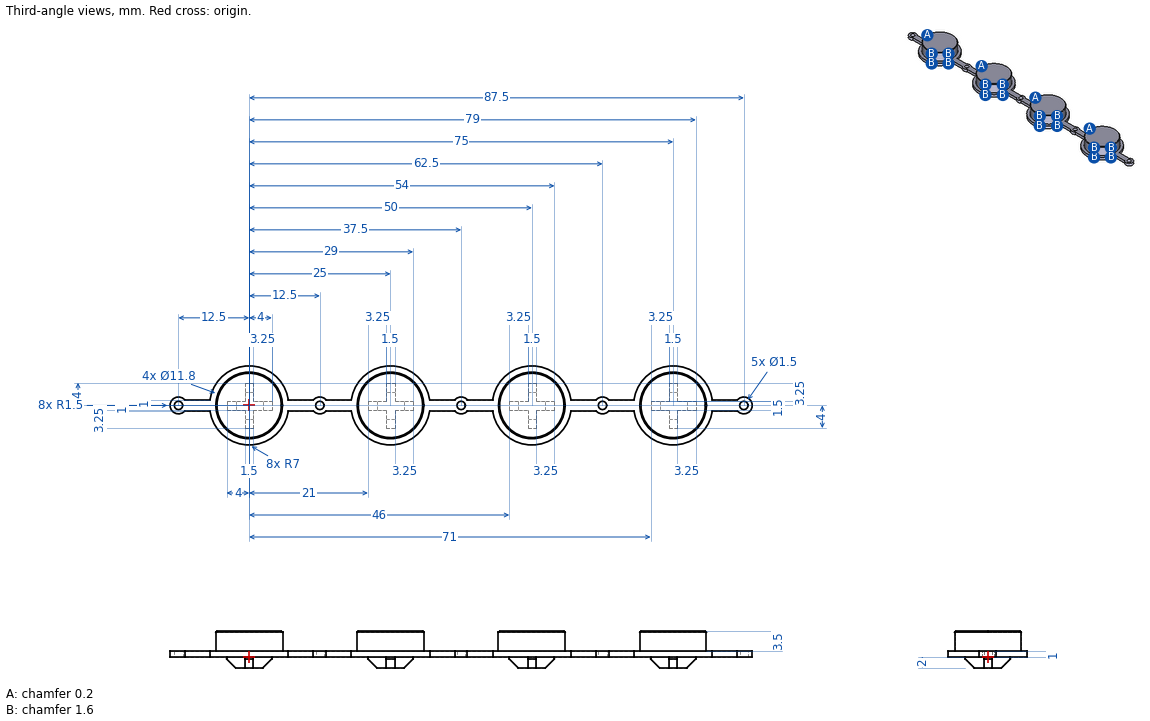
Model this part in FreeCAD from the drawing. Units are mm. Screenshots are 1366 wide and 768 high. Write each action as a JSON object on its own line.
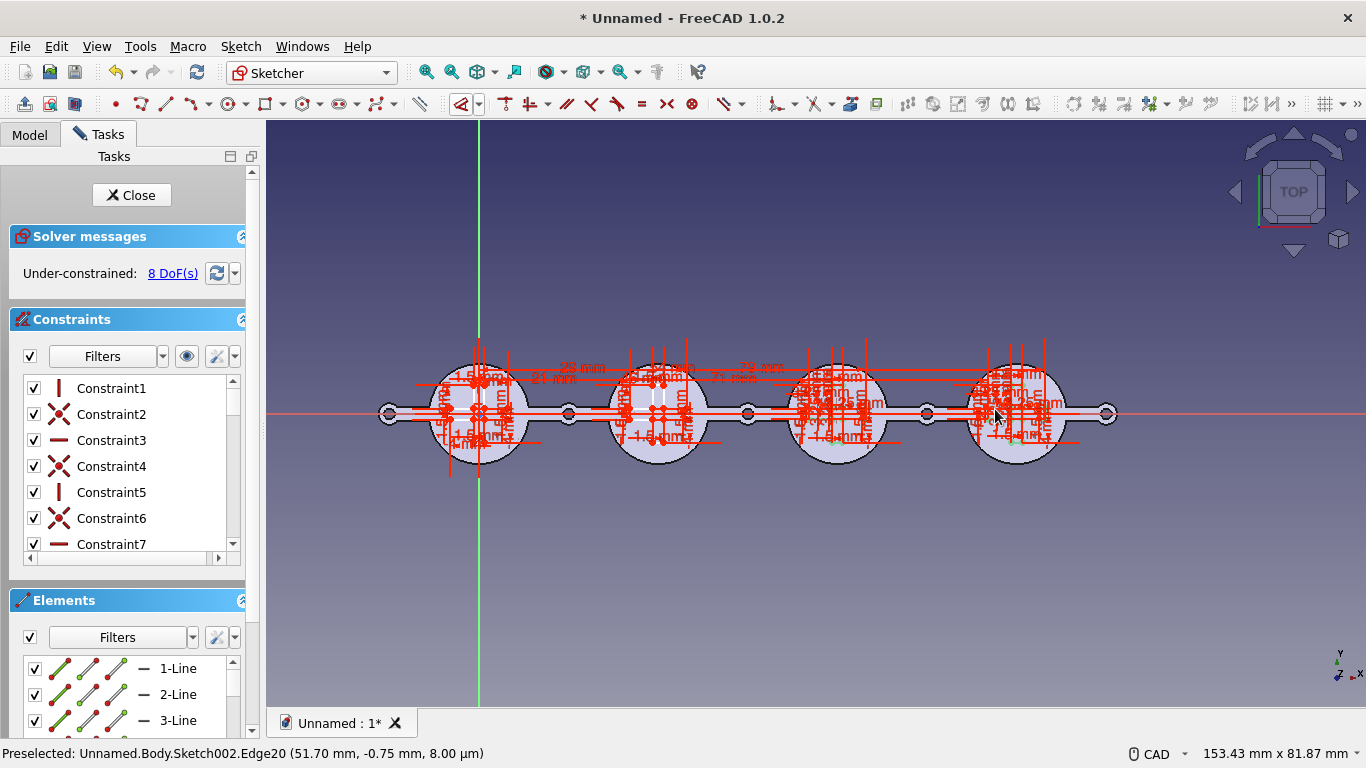
{"action": "scroll", "coordinate": [637, 409], "scroll_direction": "up", "scroll_amount": 5}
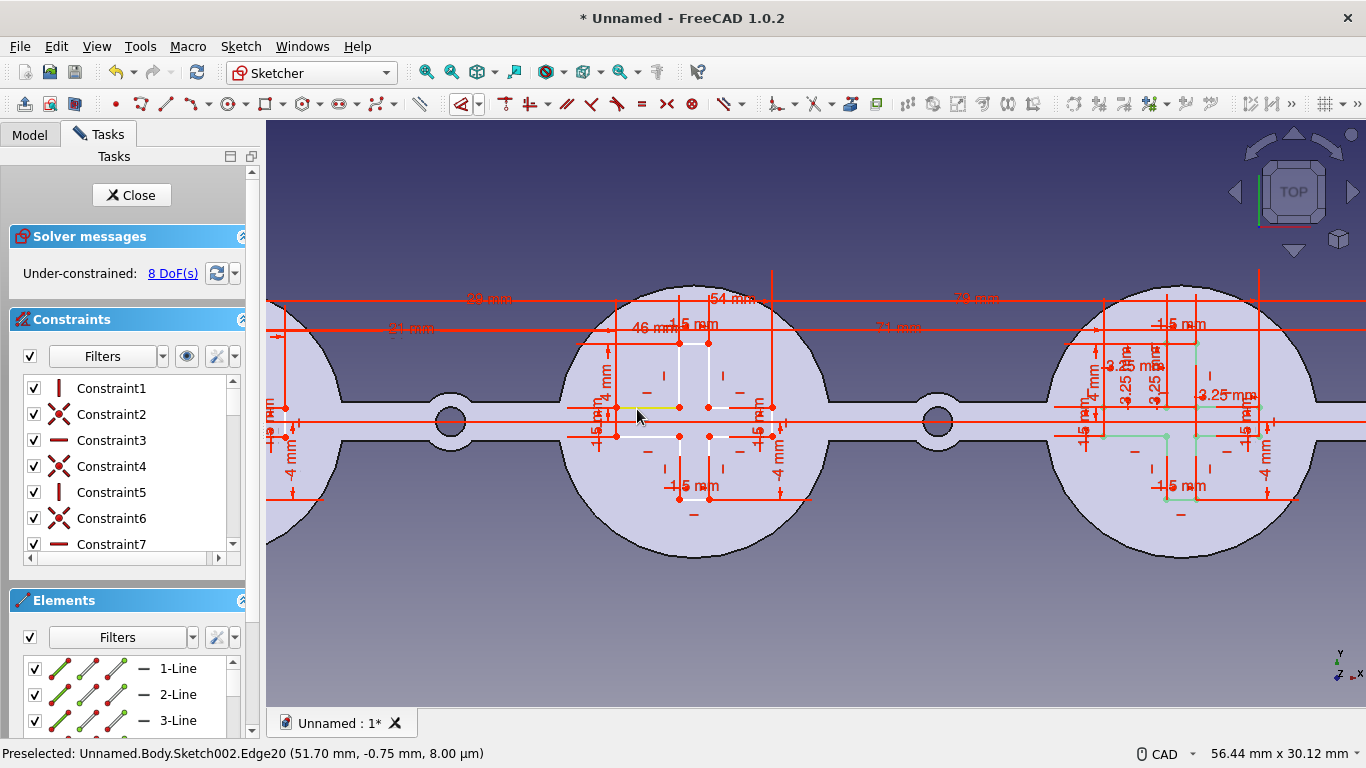
{"action": "left_click", "coordinate": [635, 408]}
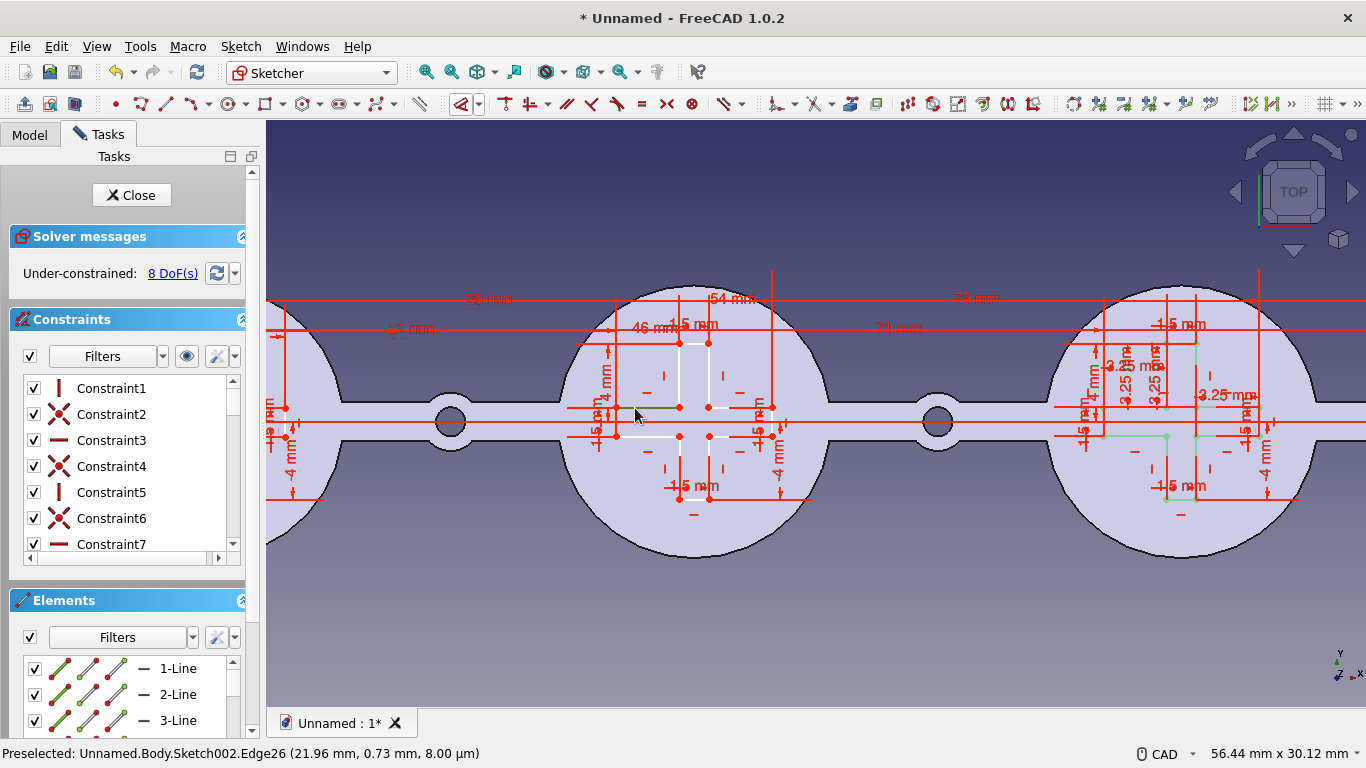
{"action": "left_click", "coordinate": [478, 104]}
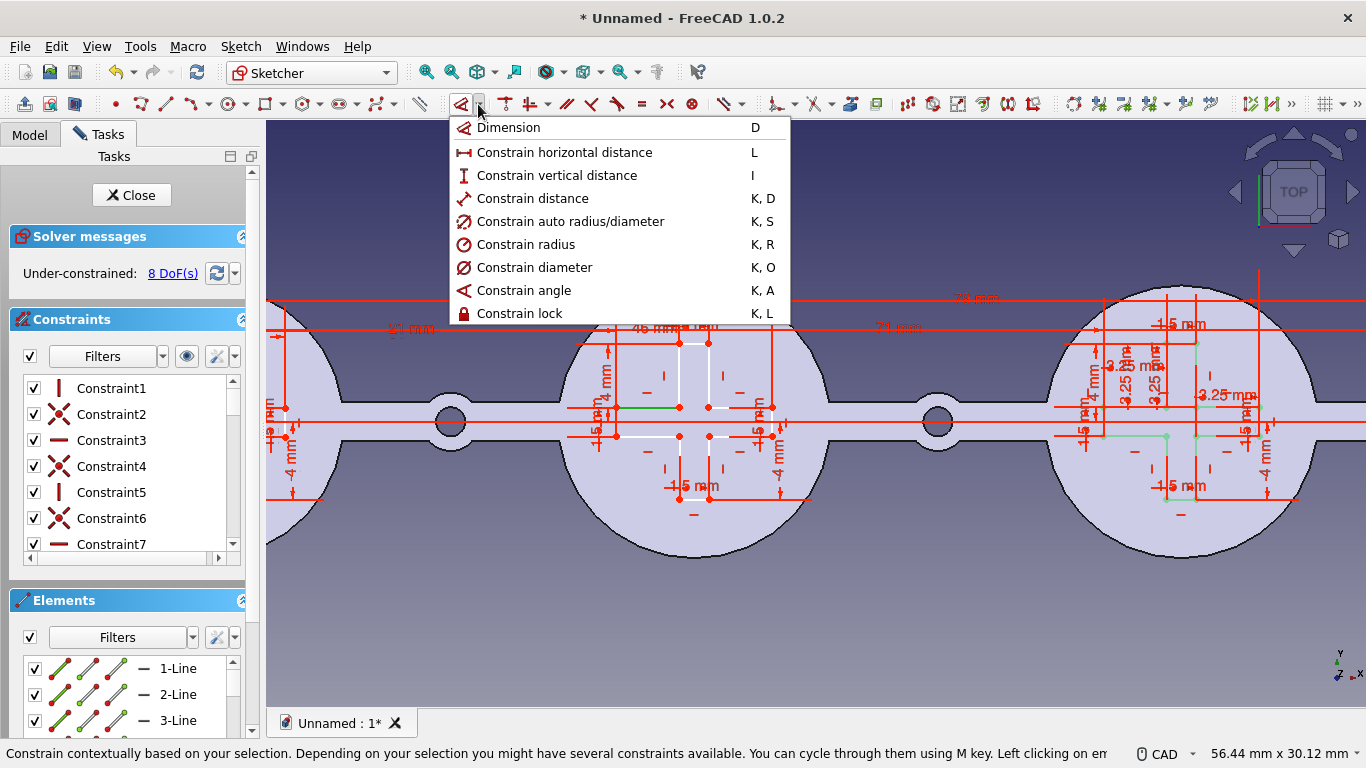
{"action": "left_click", "coordinate": [620, 152]}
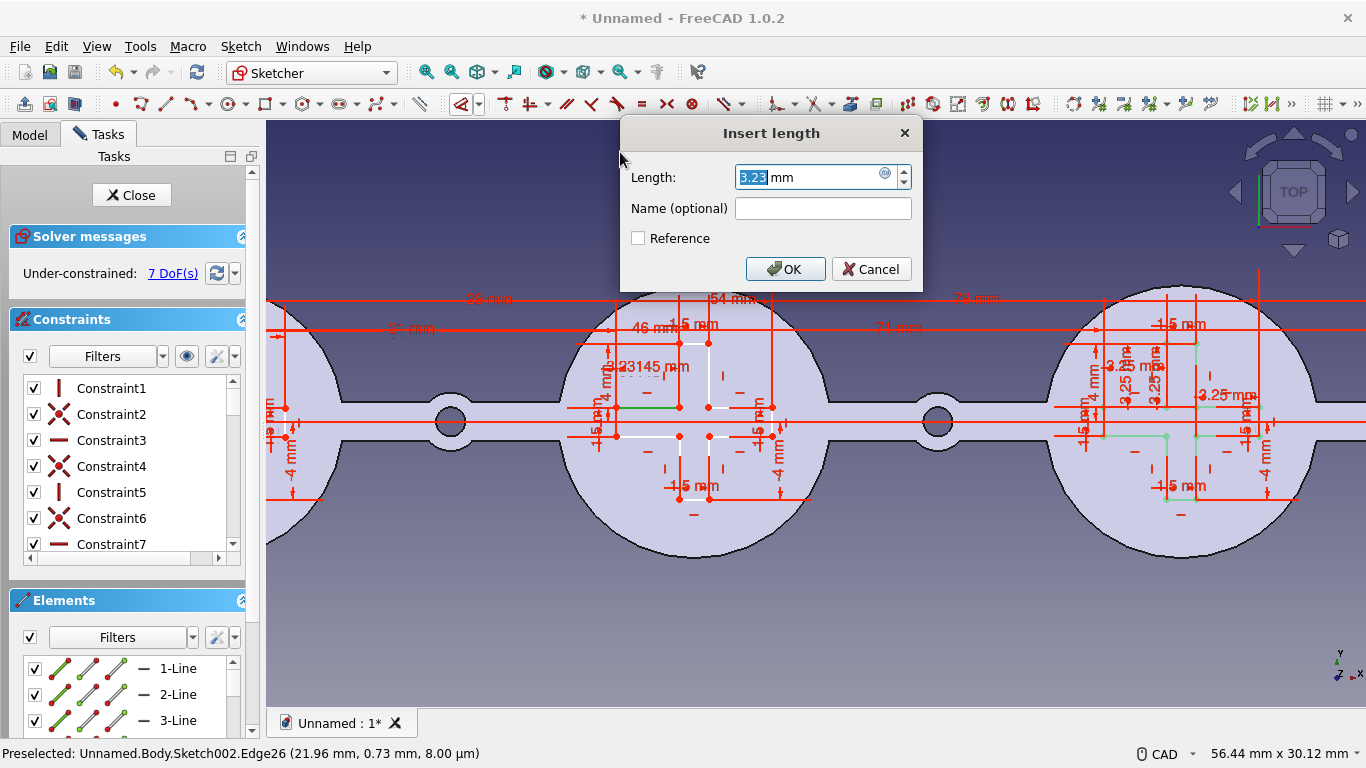
{"action": "type", "text": "3.25"}
{"action": "key", "text": "Return"}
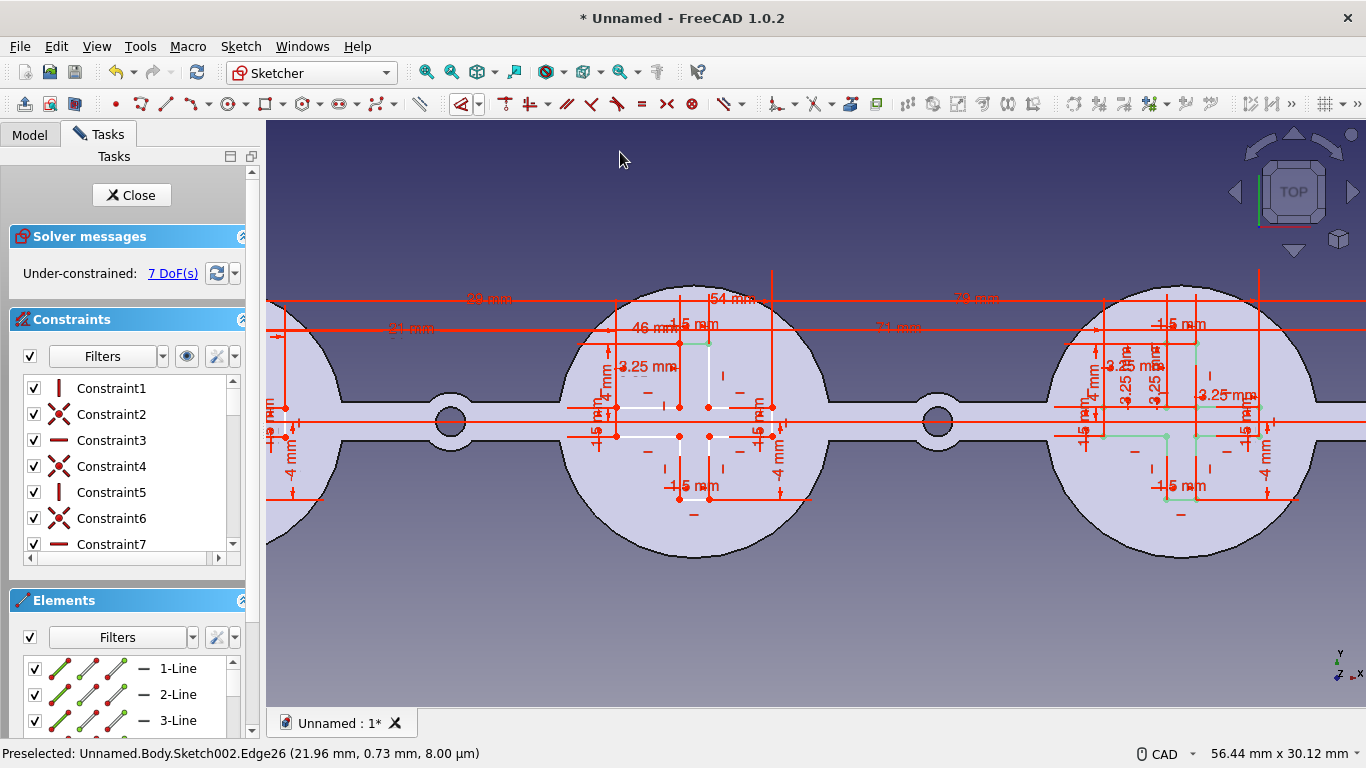
{"action": "left_click", "coordinate": [680, 389]}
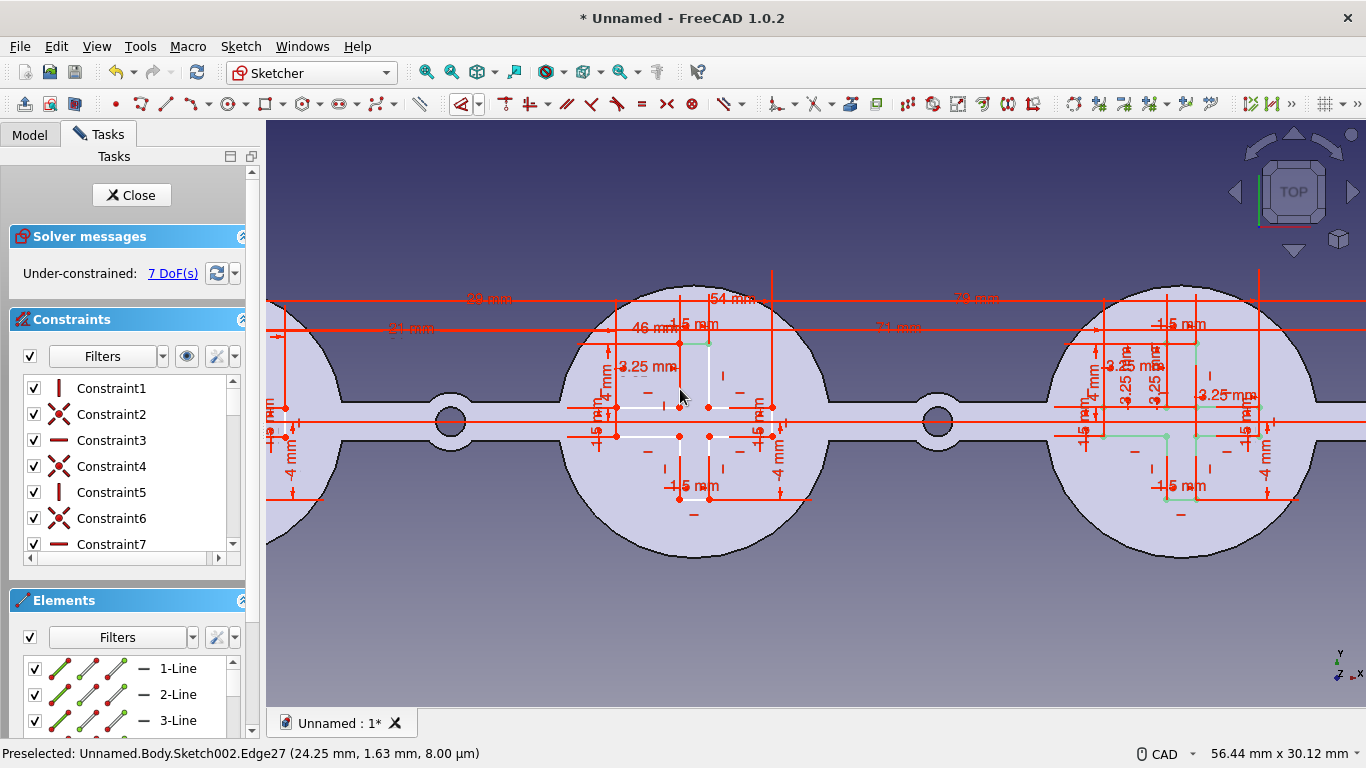
{"action": "key", "text": "i"}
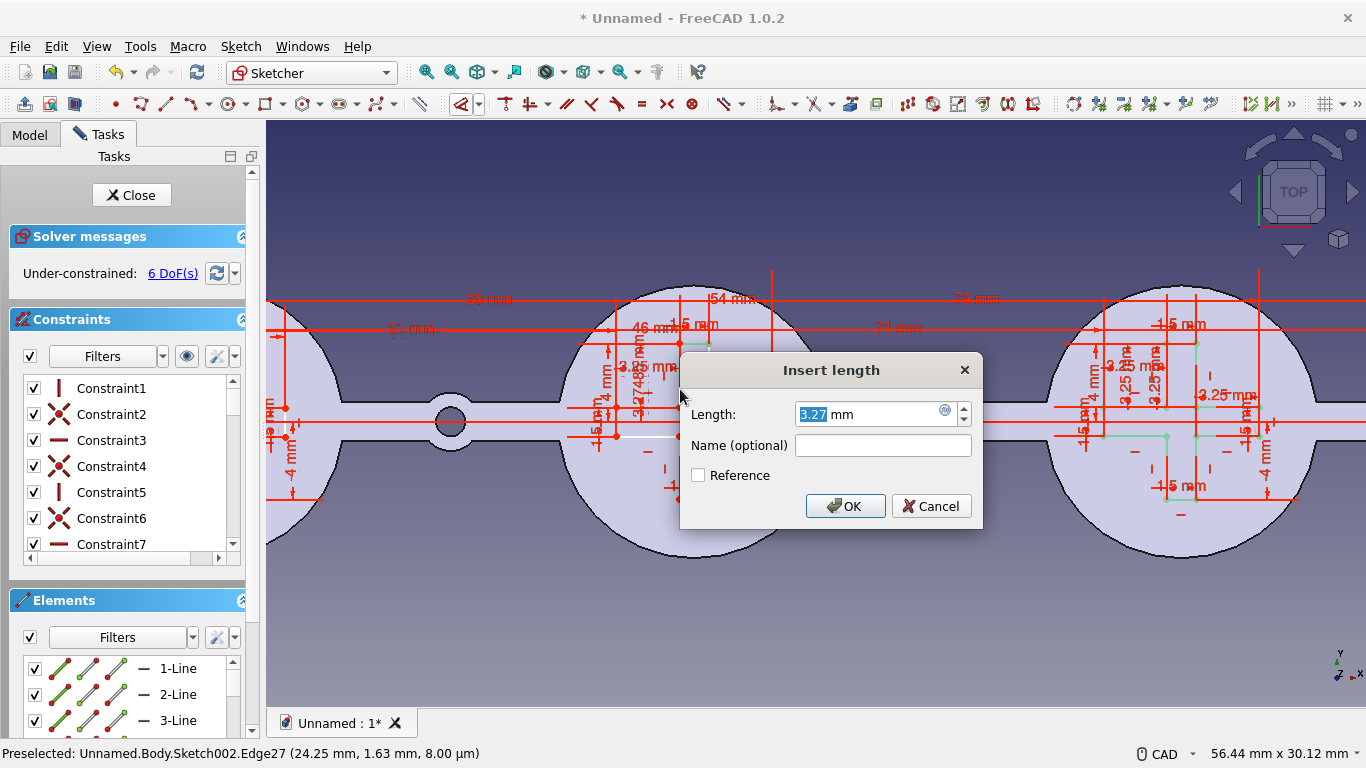
{"action": "type", "text": "3.25"}
{"action": "key", "text": "Return"}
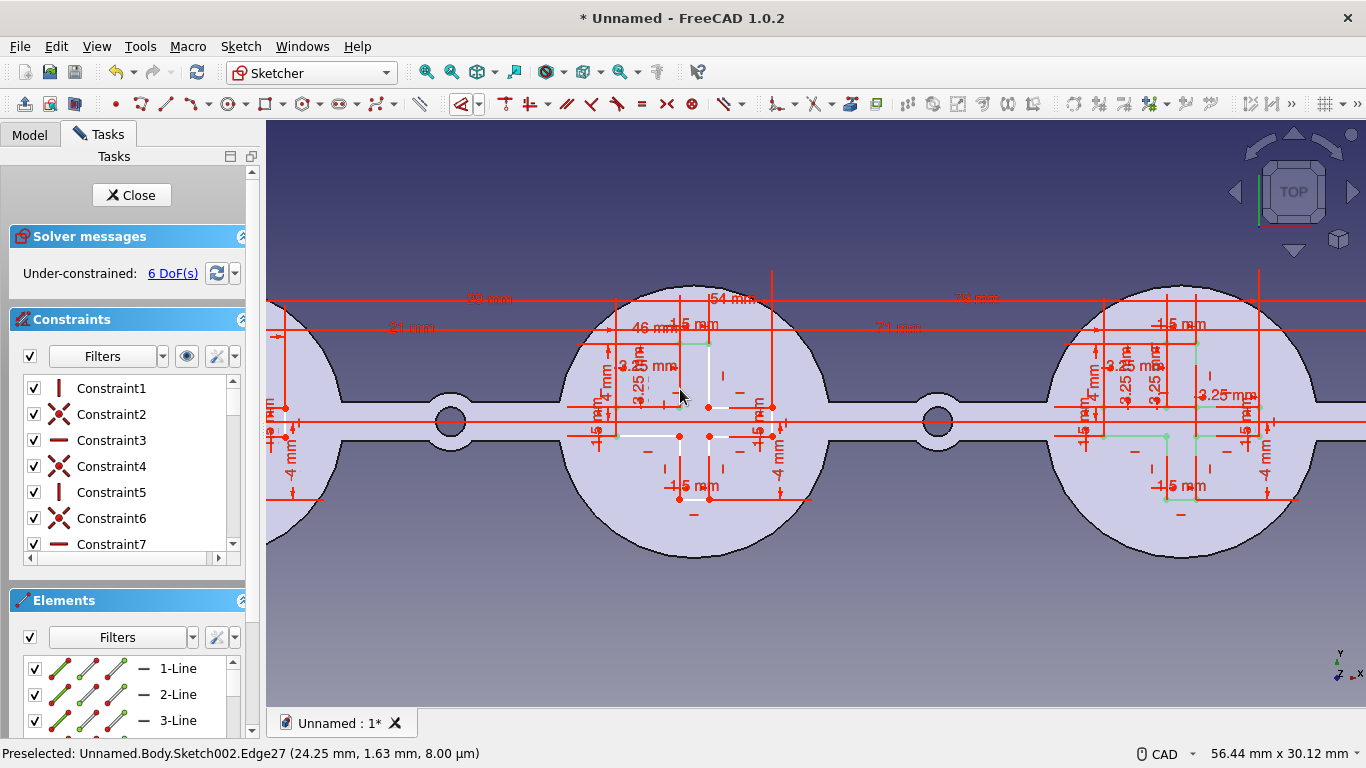
{"action": "left_click", "coordinate": [709, 363]}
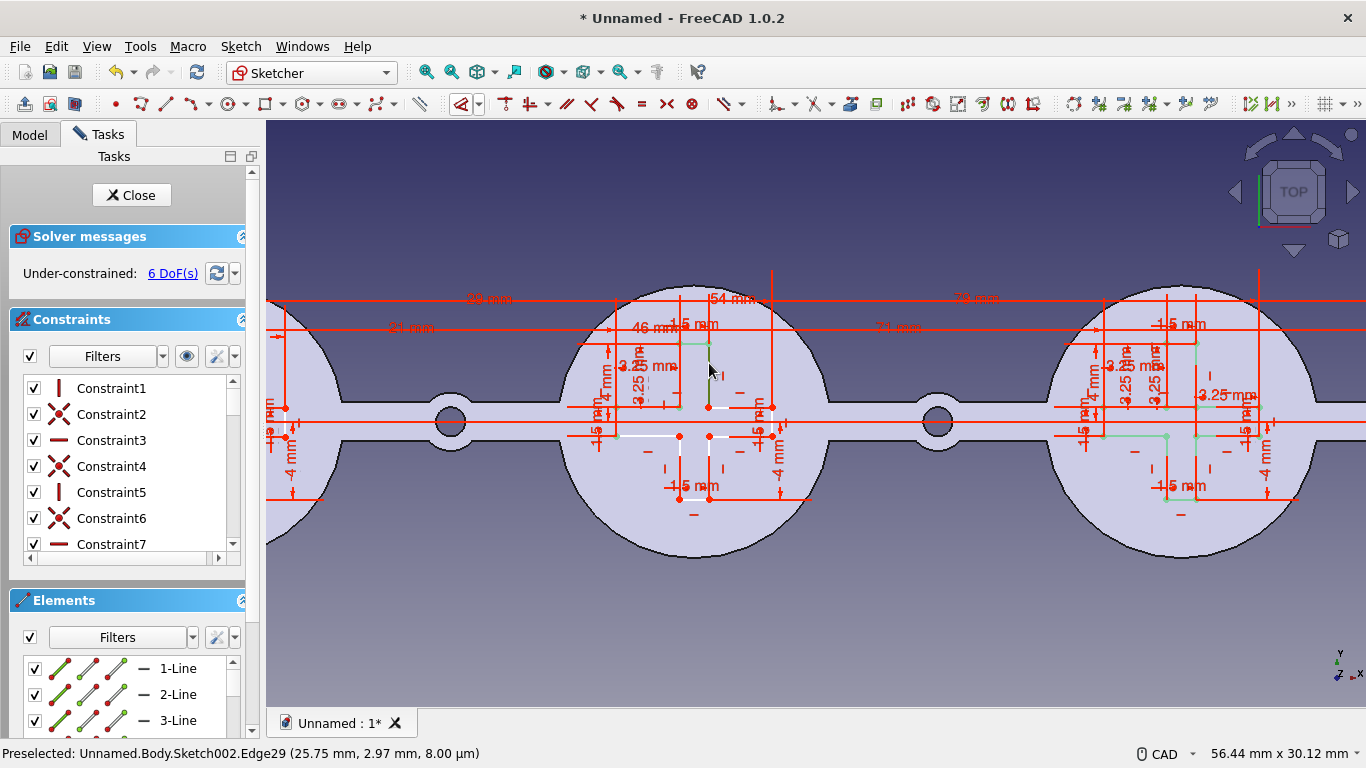
{"action": "key", "text": "i"}